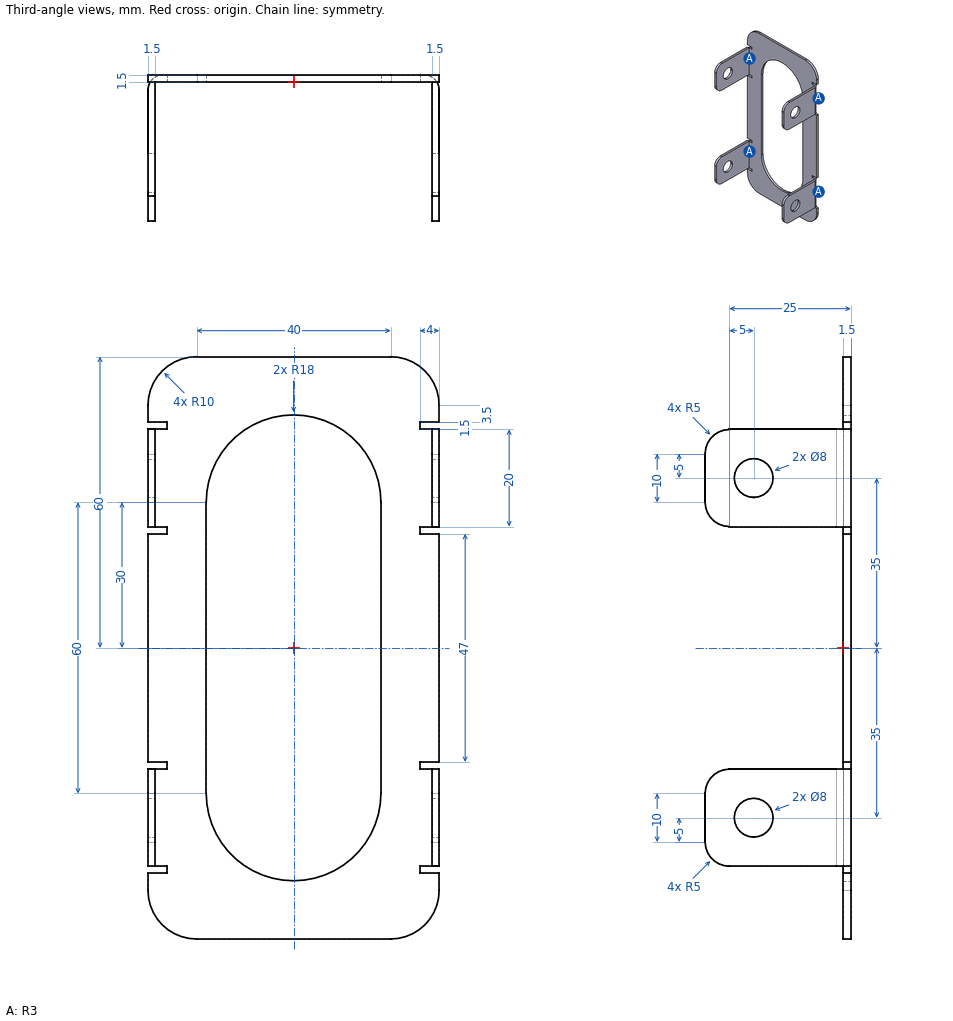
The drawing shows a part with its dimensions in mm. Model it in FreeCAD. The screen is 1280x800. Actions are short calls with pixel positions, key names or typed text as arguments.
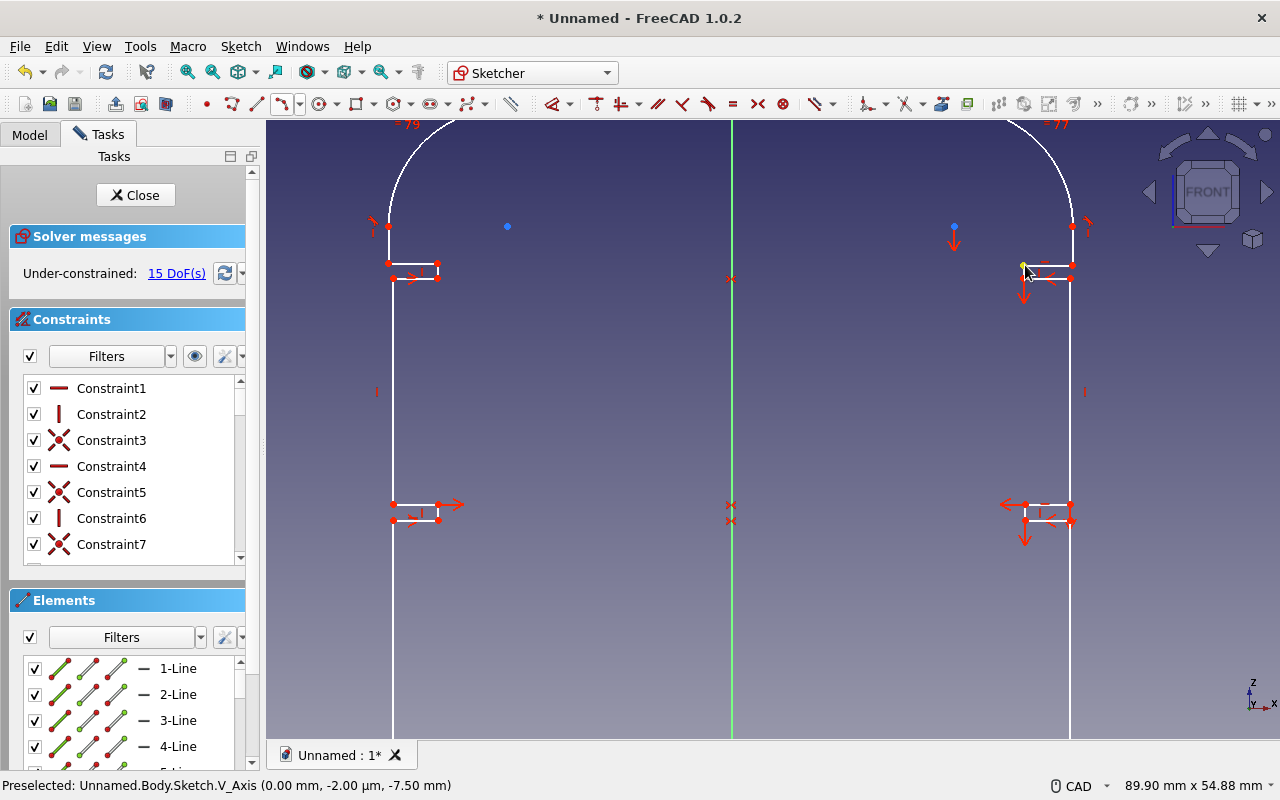
click(1024, 266)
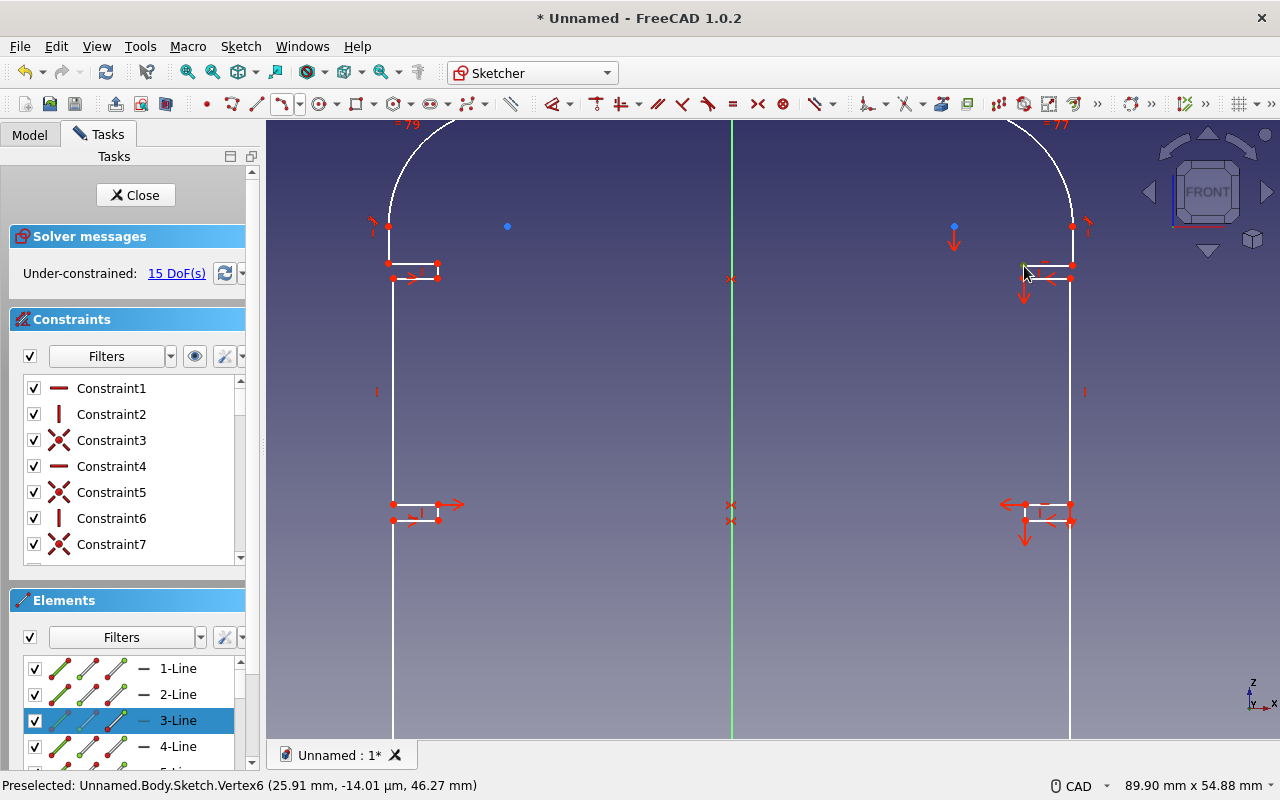
click(438, 264)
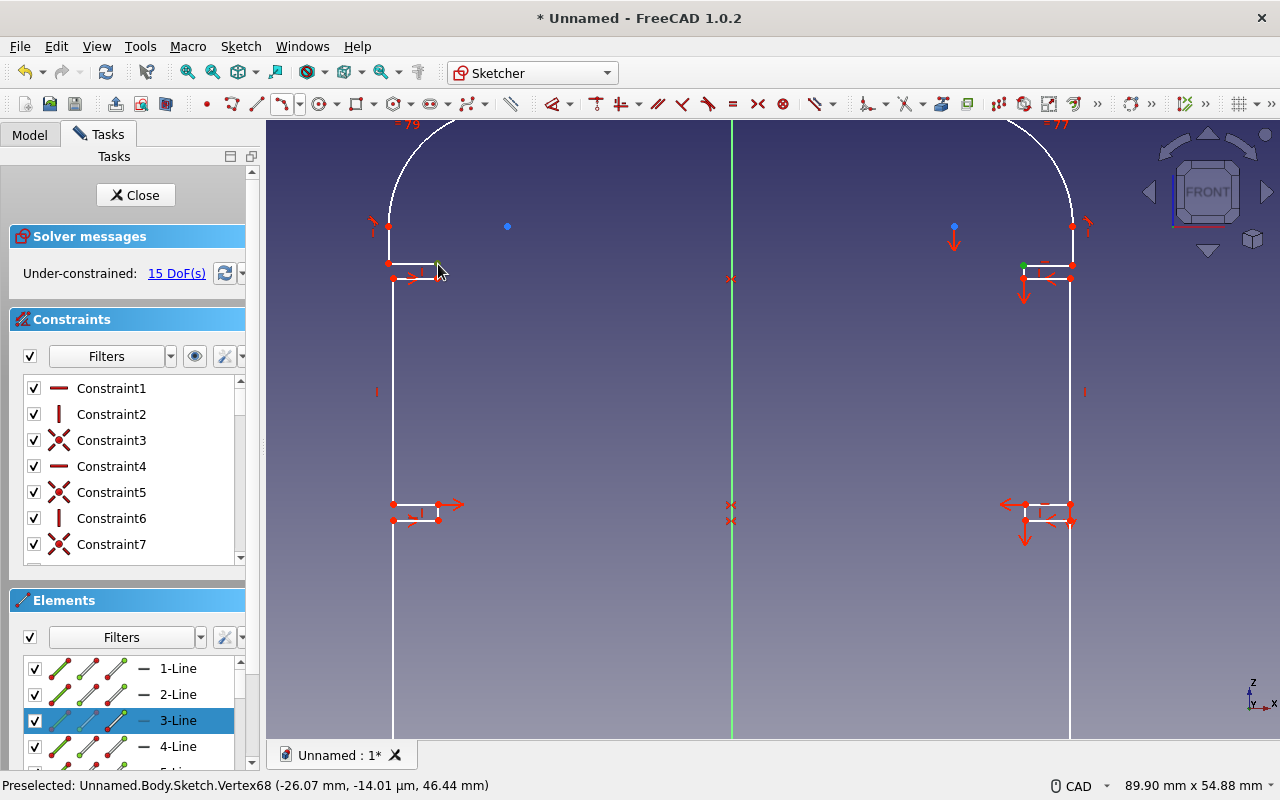
click(732, 671)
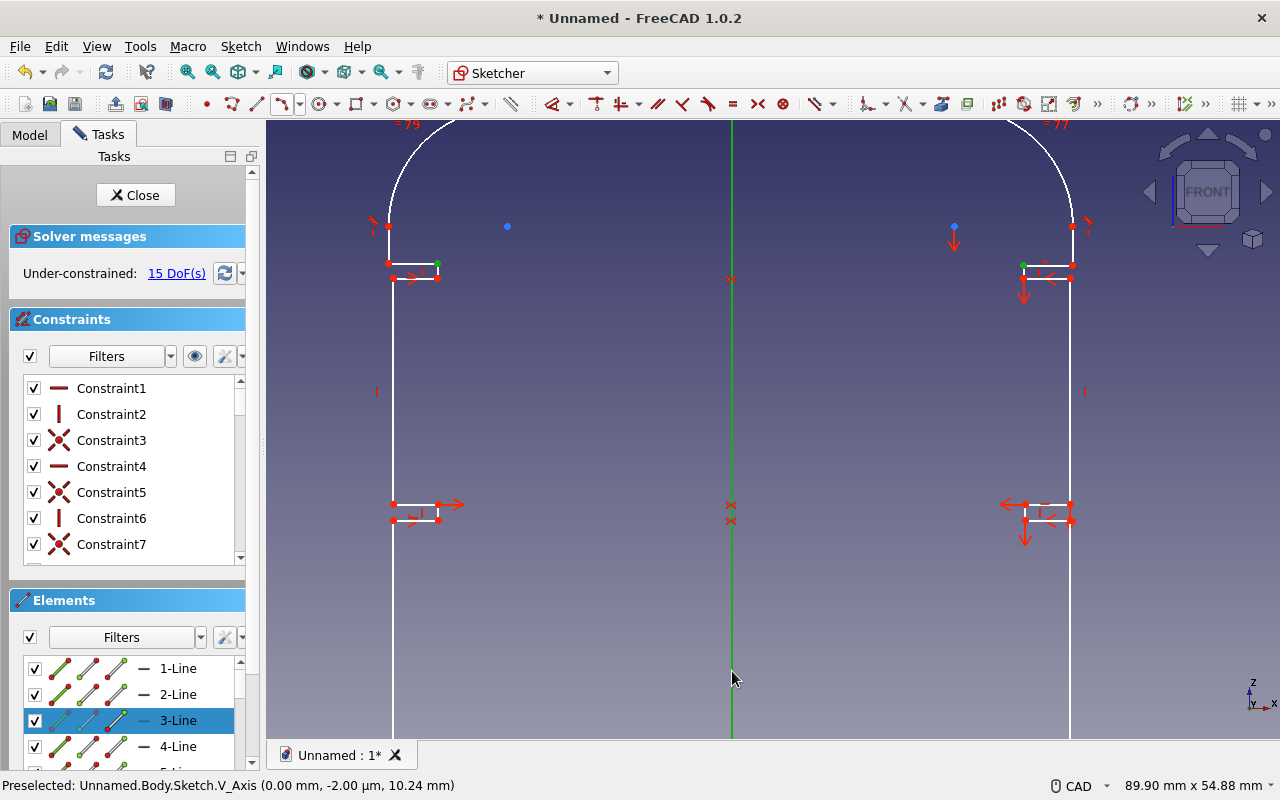
click(758, 104)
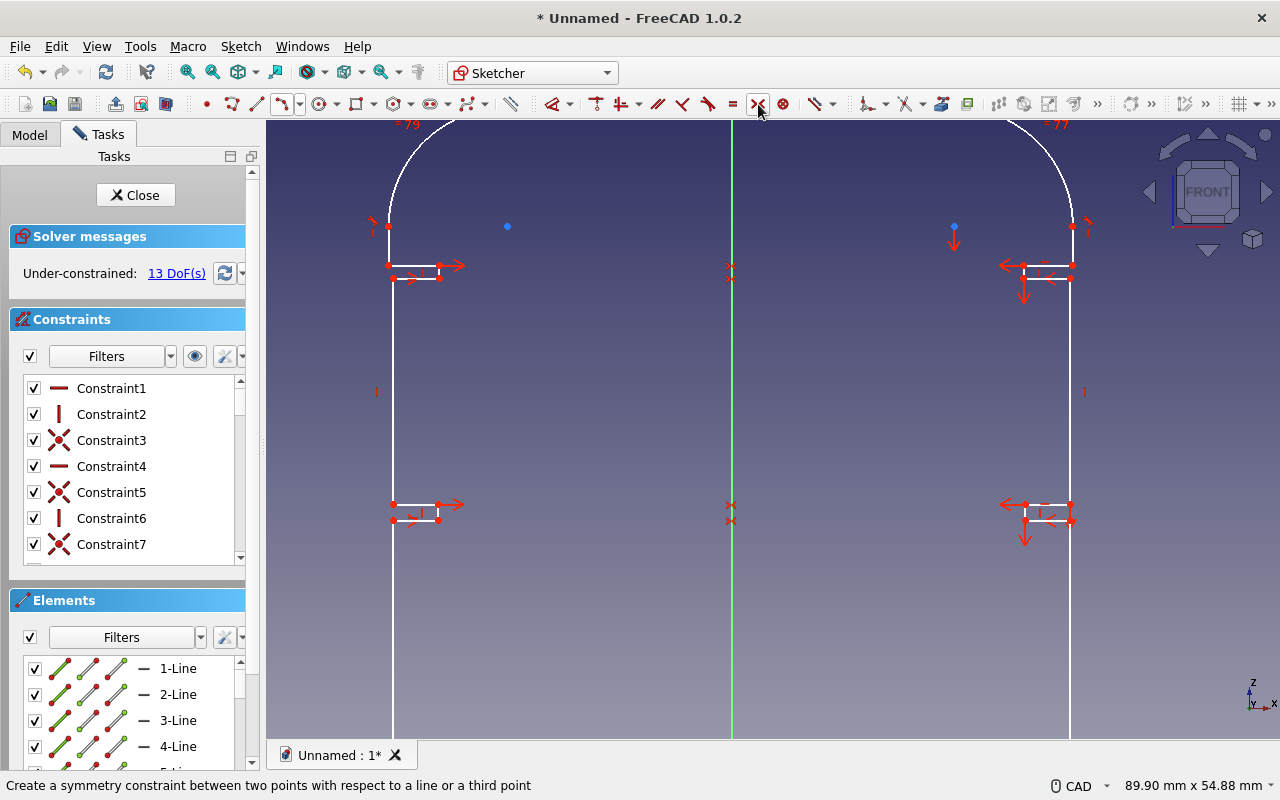
scroll(693, 275, down, 6)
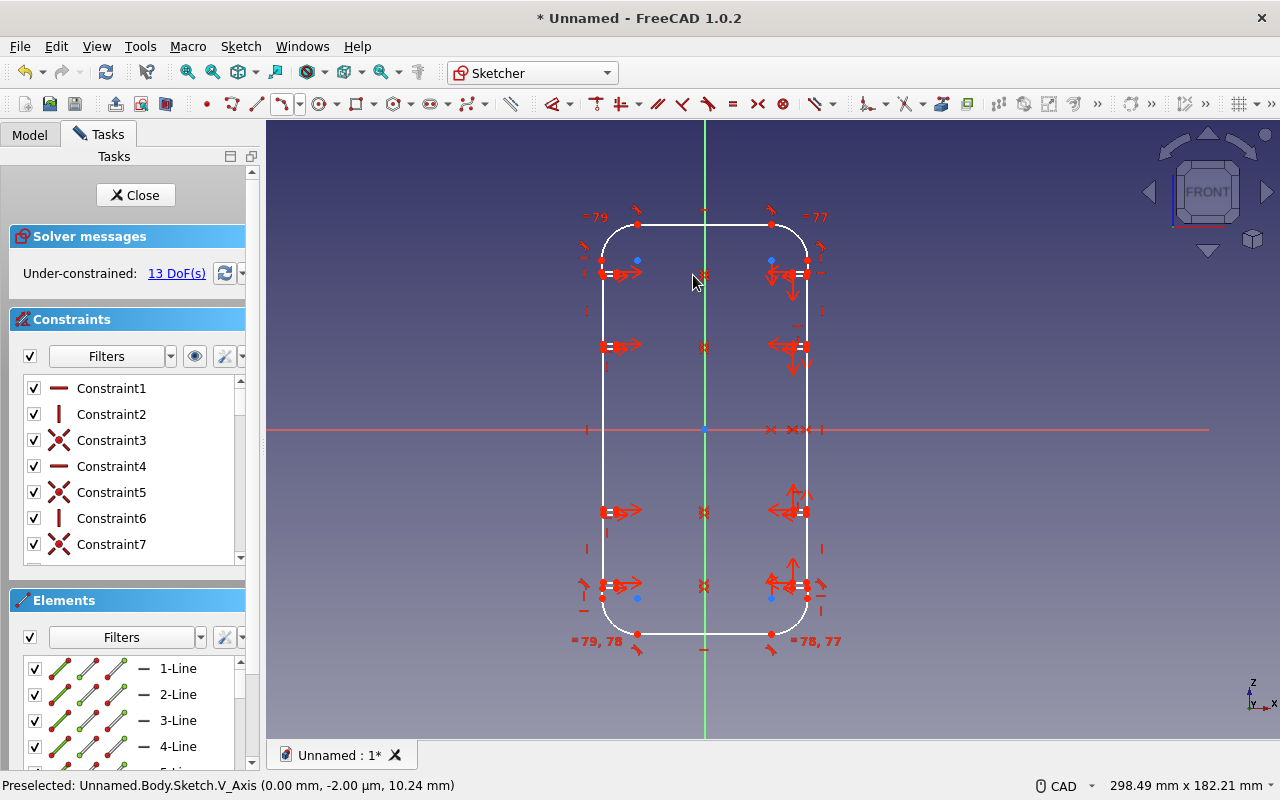
scroll(602, 588, up, 5)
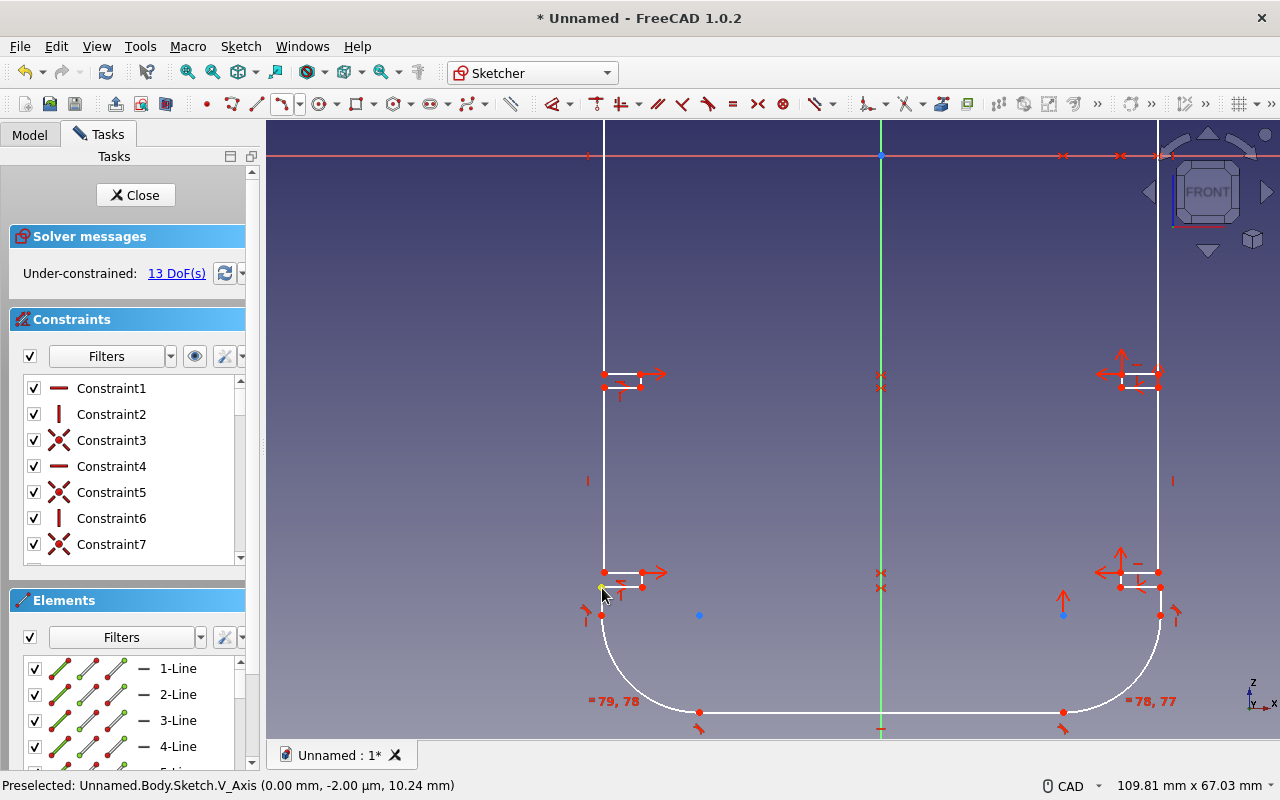
click(602, 587)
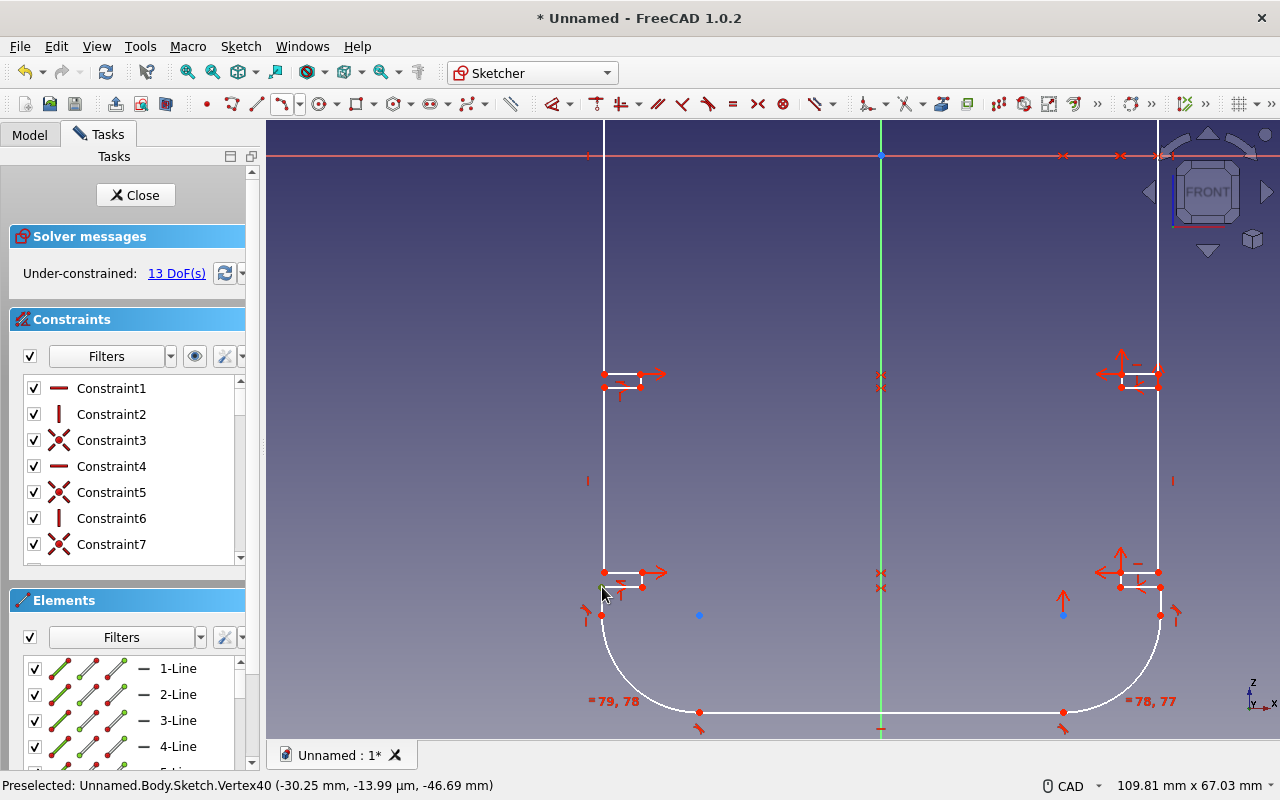
scroll(602, 589, down, 5)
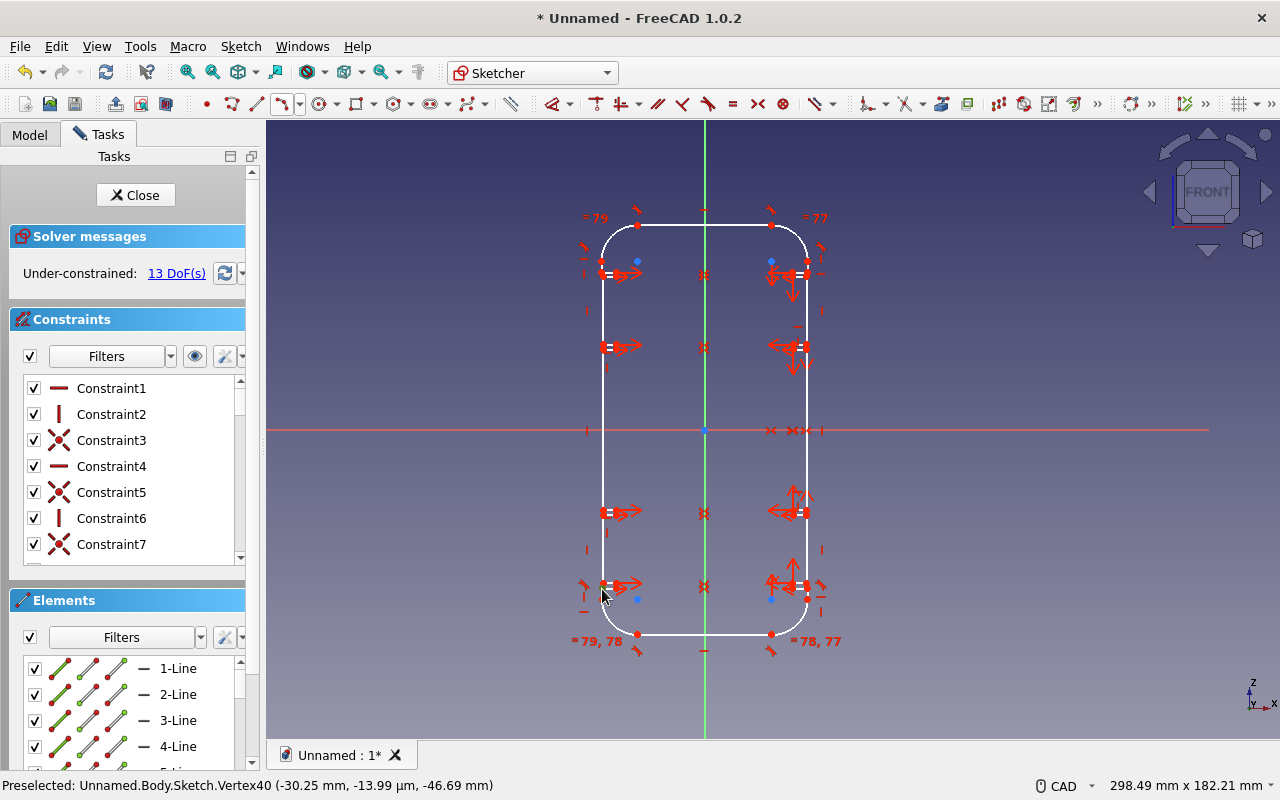
scroll(602, 273, up, 6)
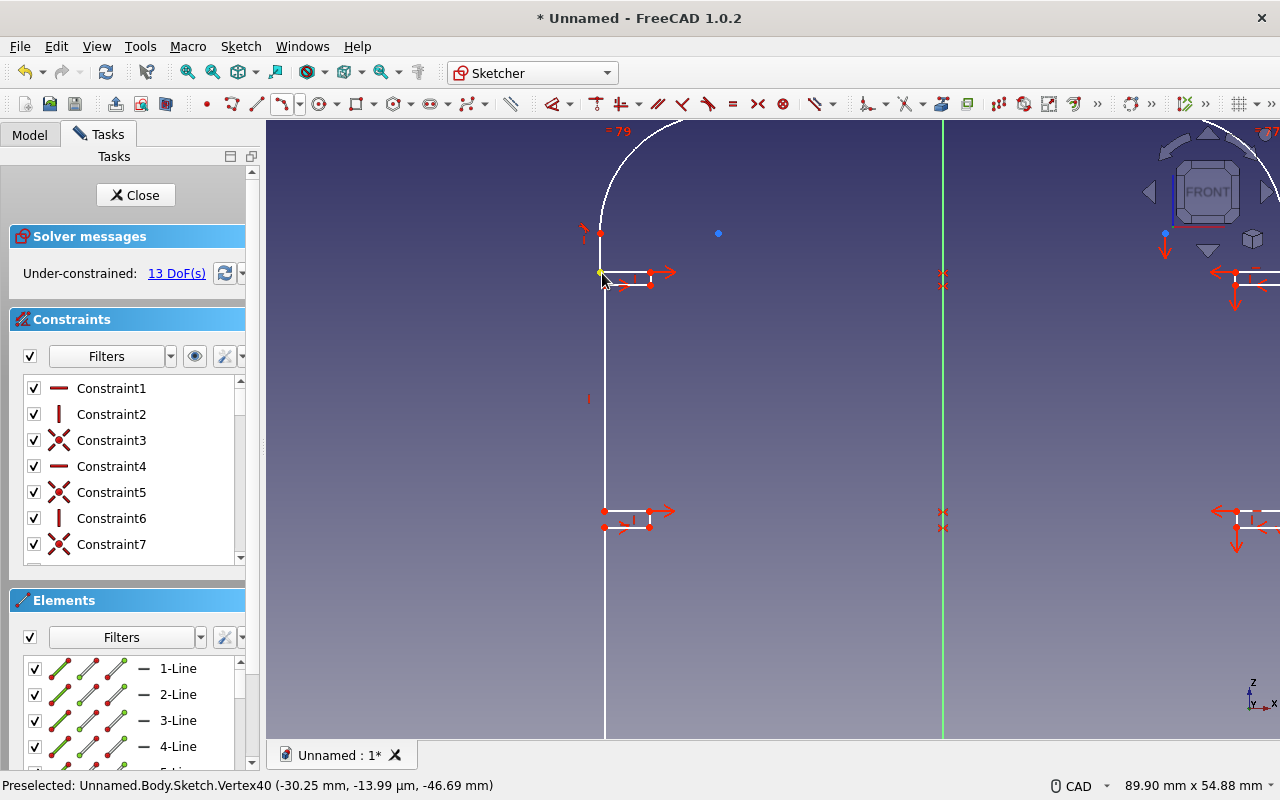
click(600, 272)